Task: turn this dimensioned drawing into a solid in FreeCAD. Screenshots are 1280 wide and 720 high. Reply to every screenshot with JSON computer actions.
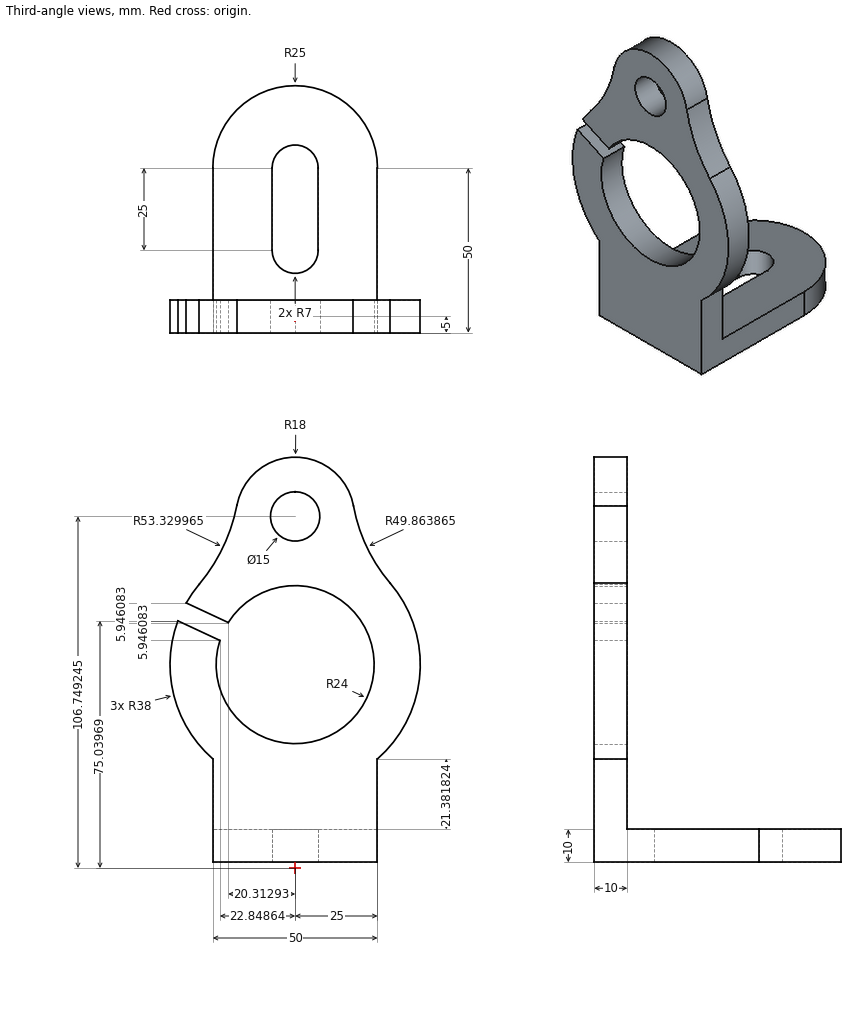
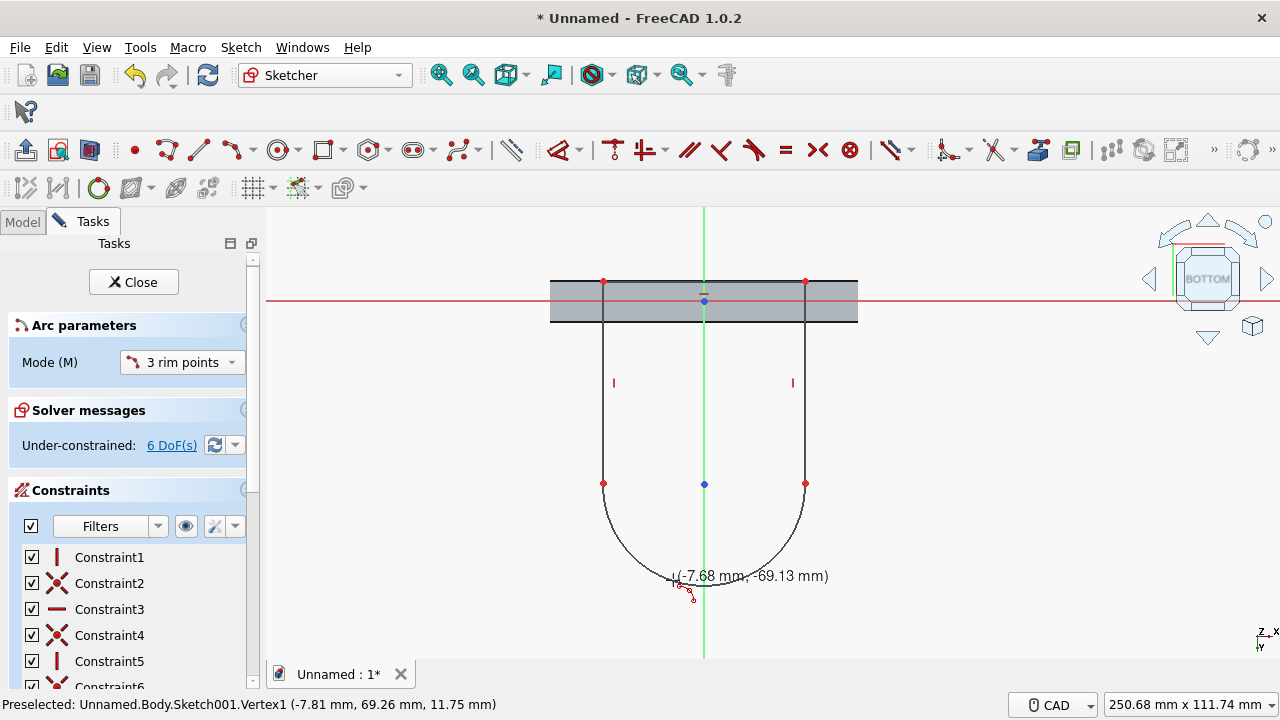
{"action": "left_click", "coordinate": [414, 150]}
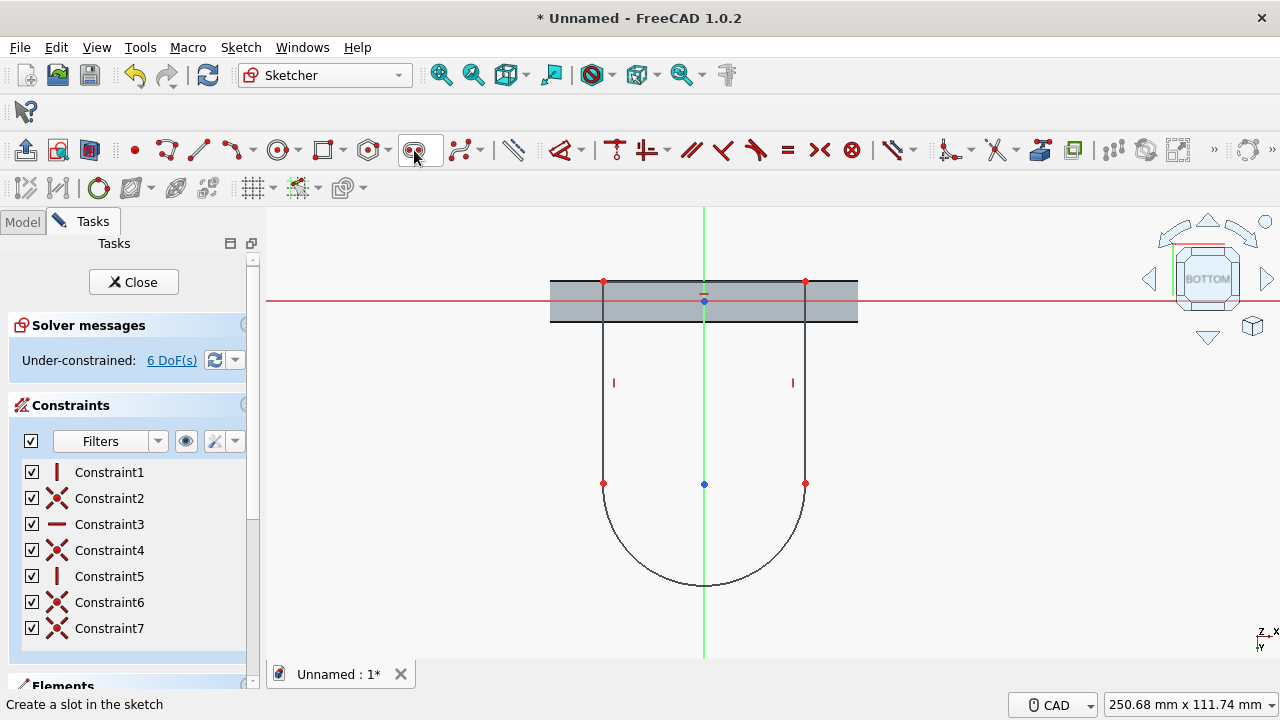
{"action": "left_click", "coordinate": [704, 483]}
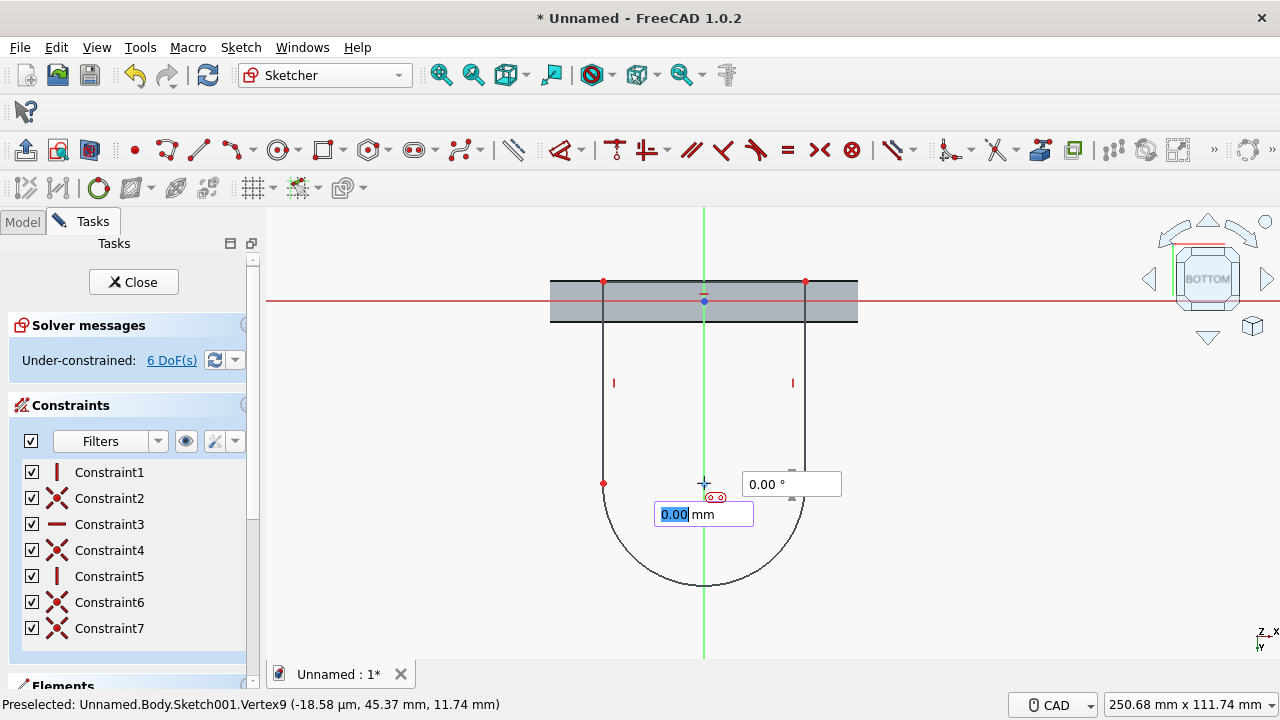
{"action": "left_click", "coordinate": [713, 382]}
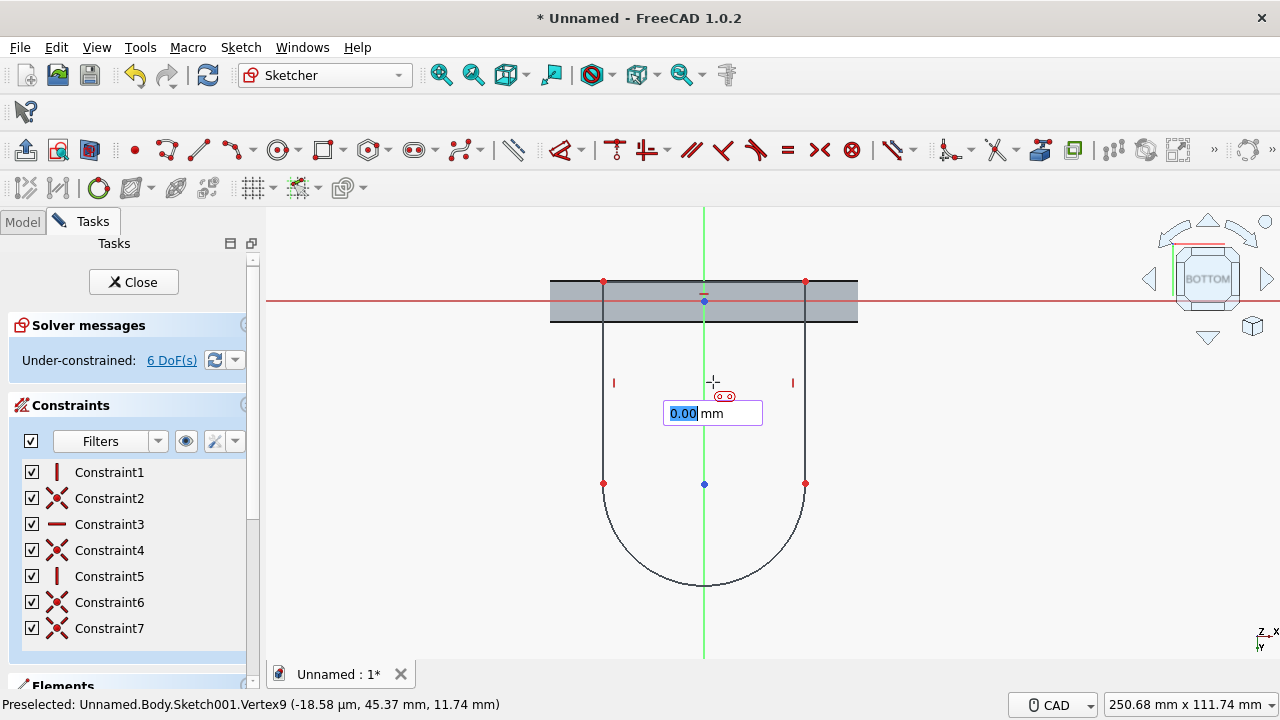
{"action": "left_click", "coordinate": [676, 433]}
{"action": "key", "text": "Escape"}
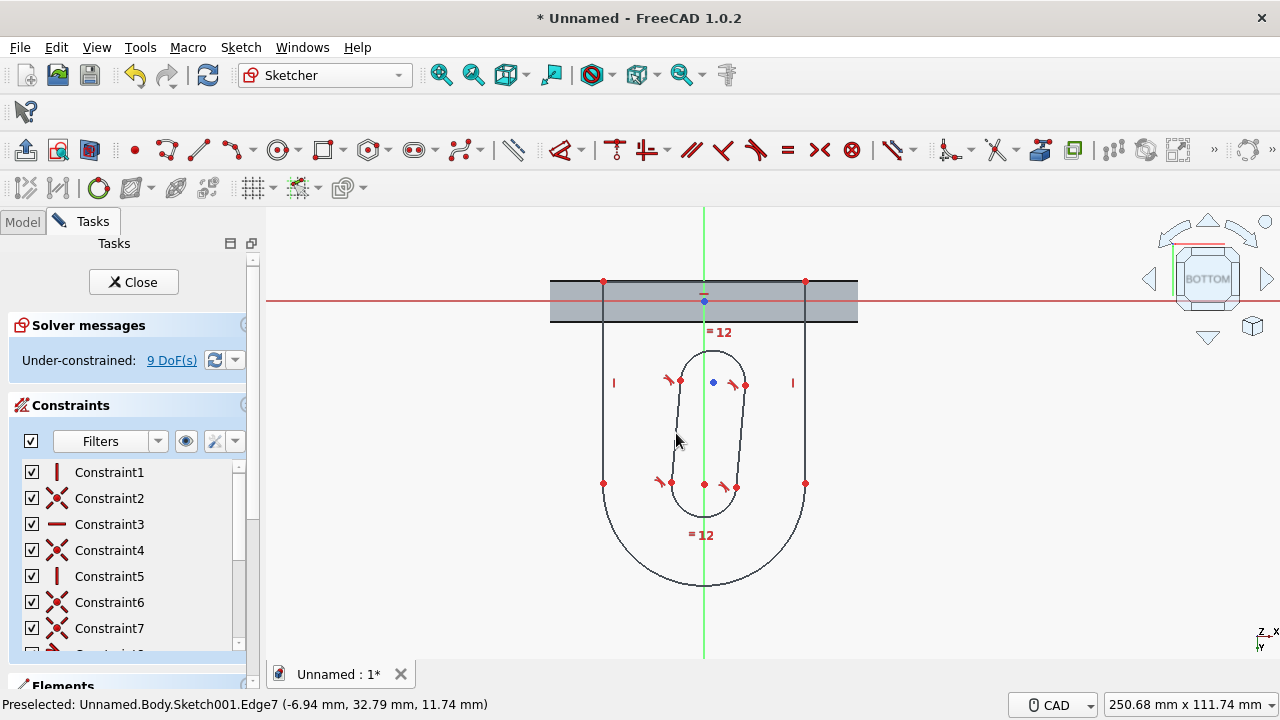
{"action": "left_click", "coordinate": [805, 423]}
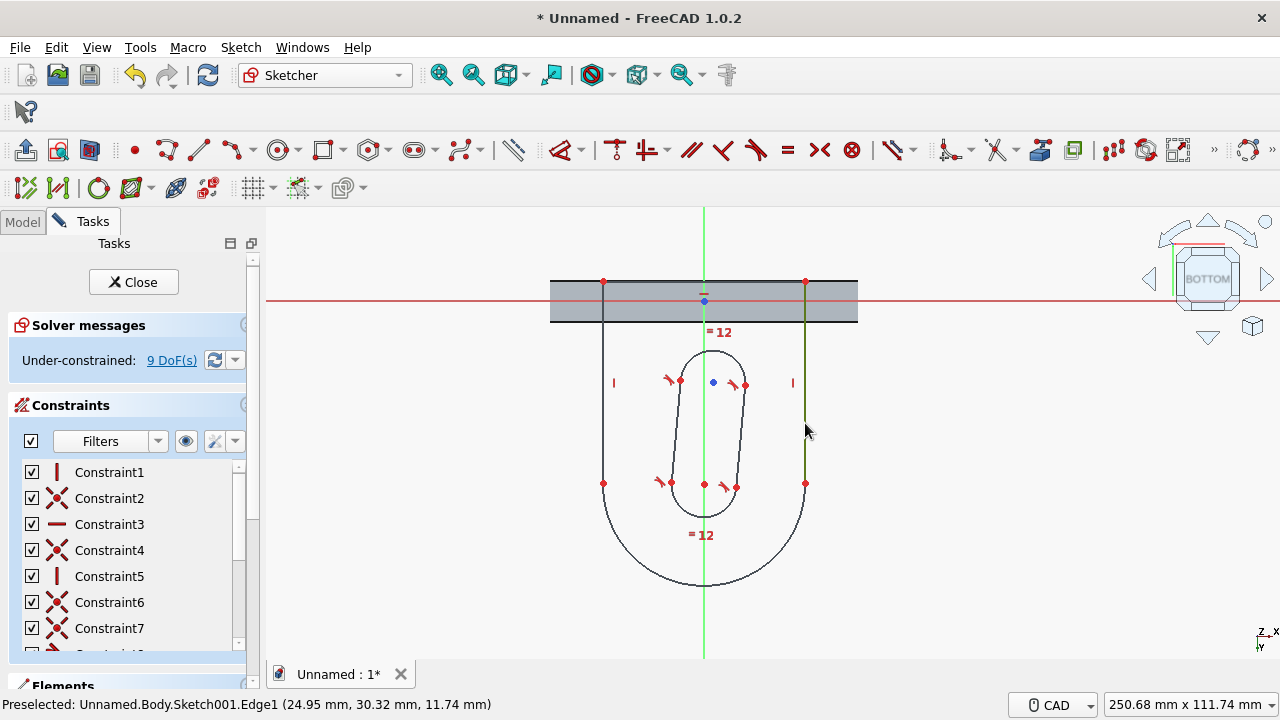
{"action": "left_click", "coordinate": [644, 566]}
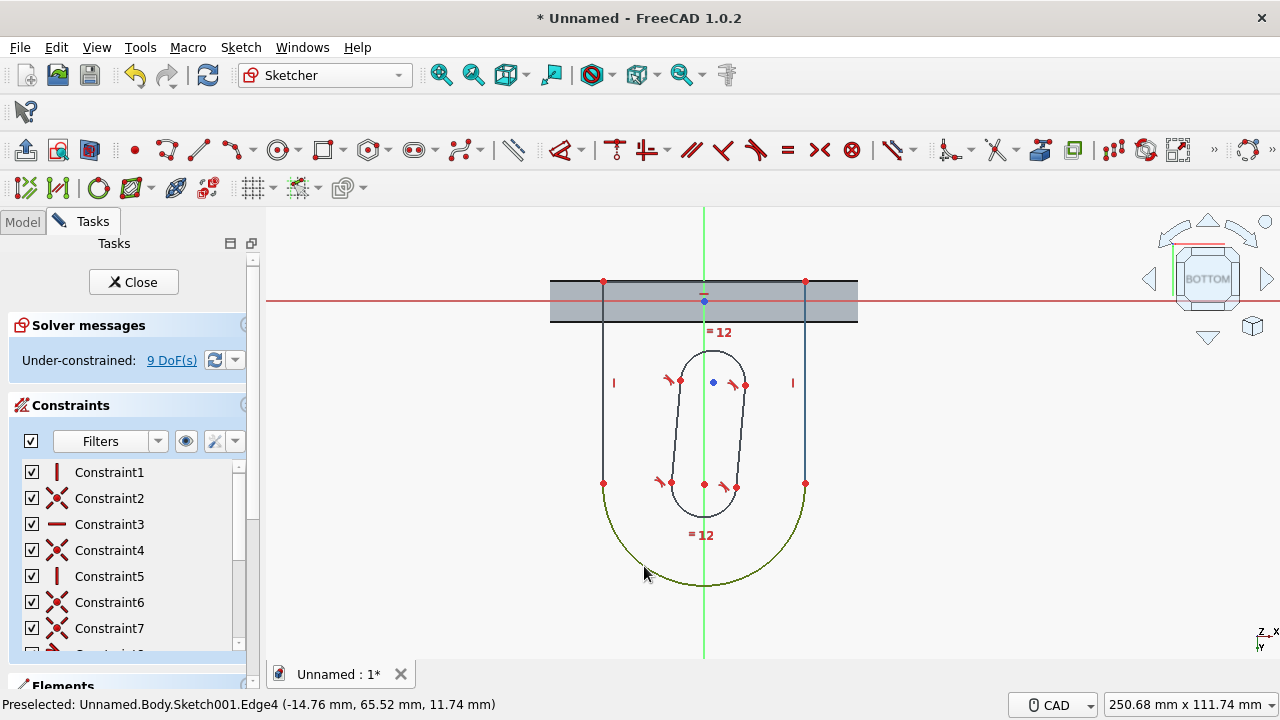
{"action": "left_click", "coordinate": [756, 150]}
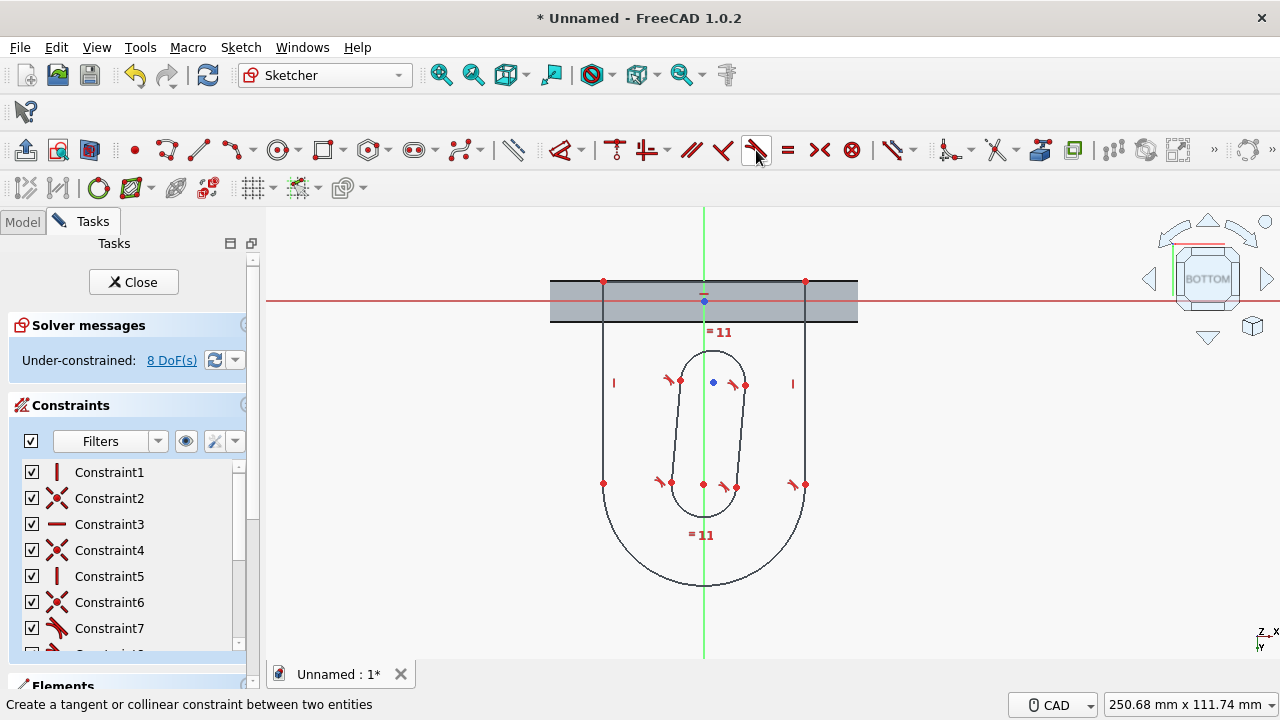
{"action": "left_click", "coordinate": [603, 343]}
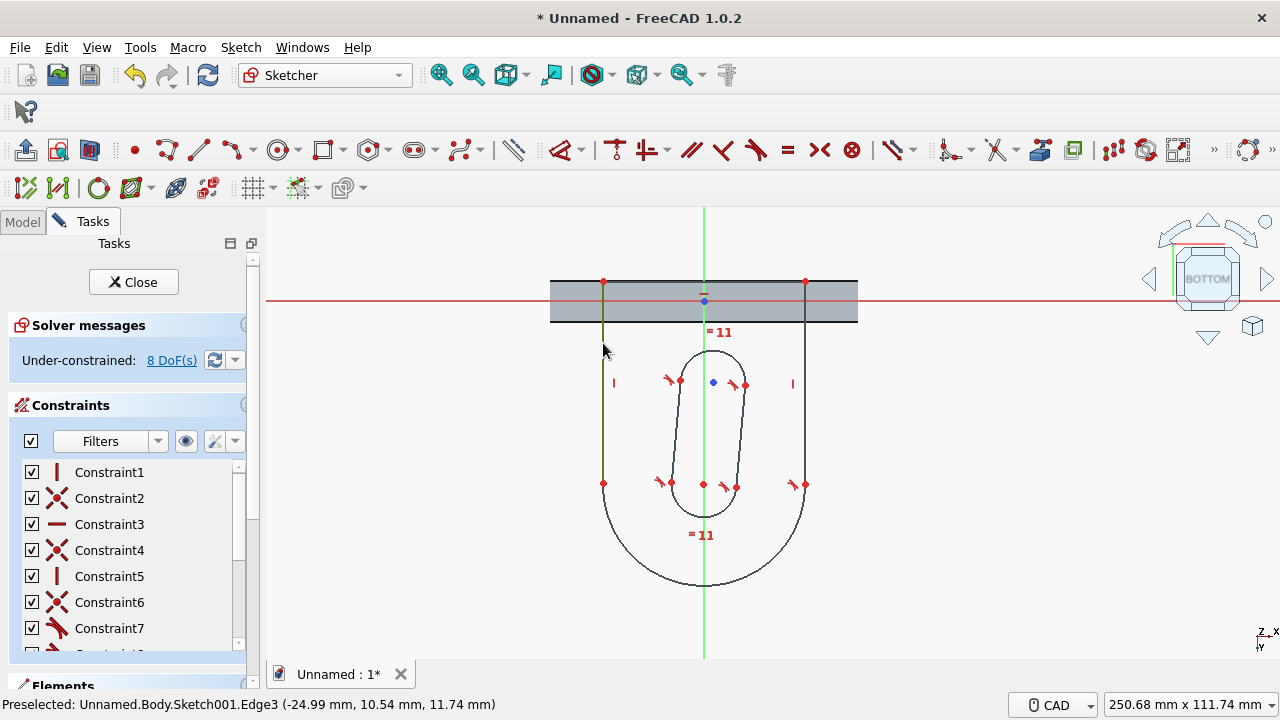
{"action": "left_click", "coordinate": [644, 566]}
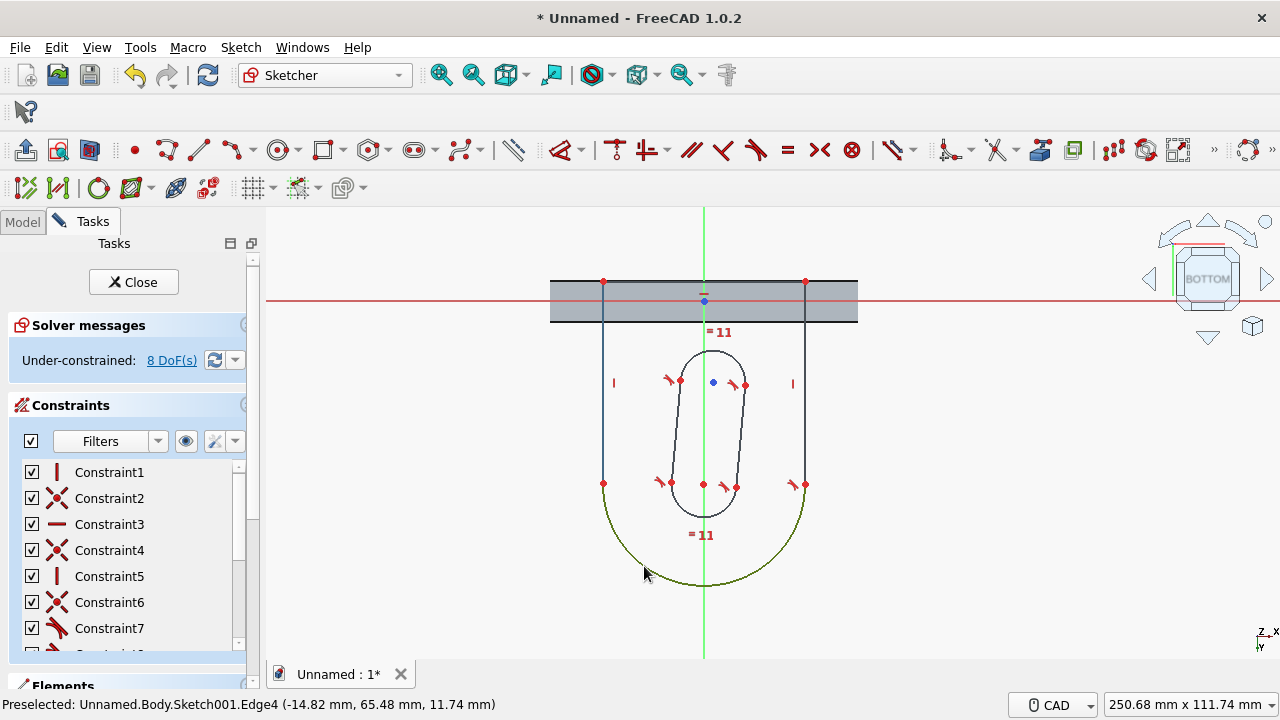
{"action": "key", "text": "t"}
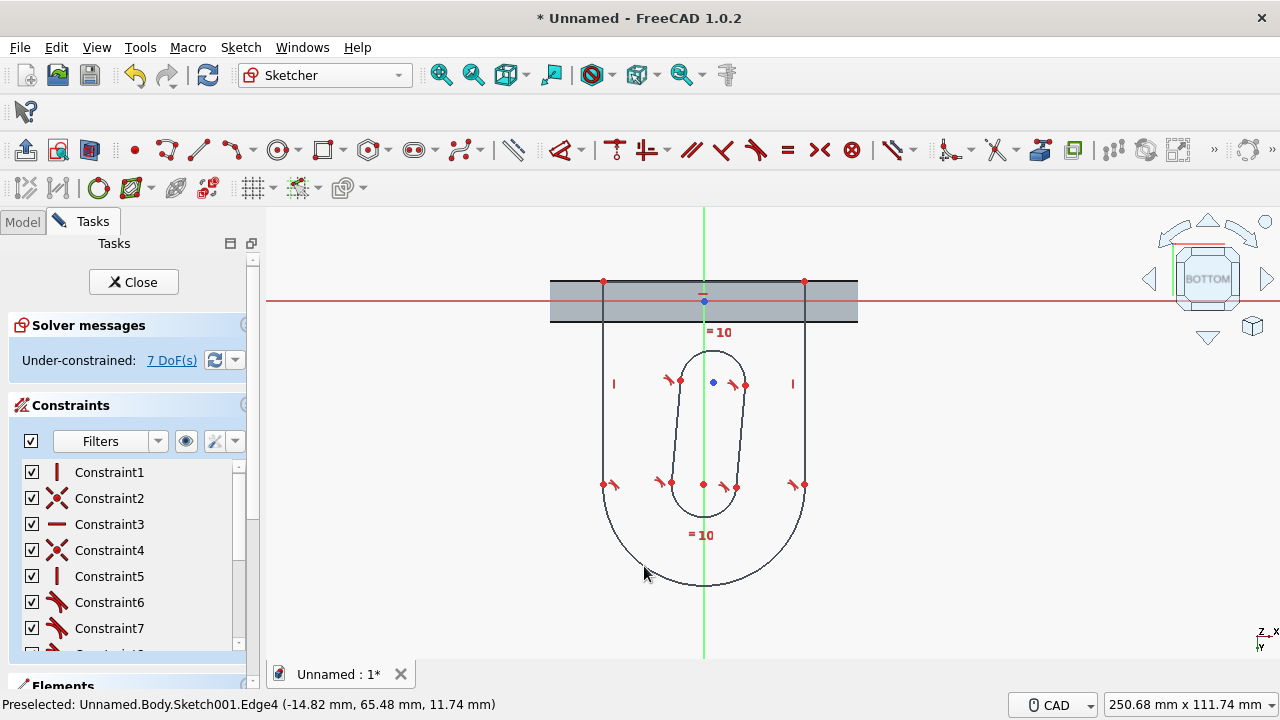
{"action": "left_click", "coordinate": [674, 451]}